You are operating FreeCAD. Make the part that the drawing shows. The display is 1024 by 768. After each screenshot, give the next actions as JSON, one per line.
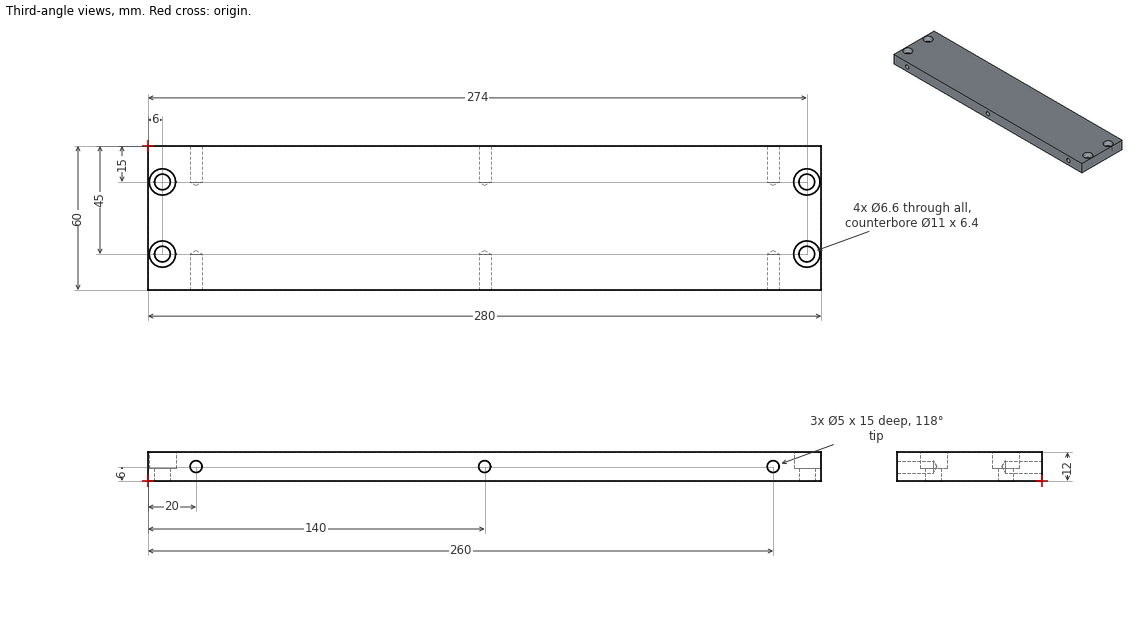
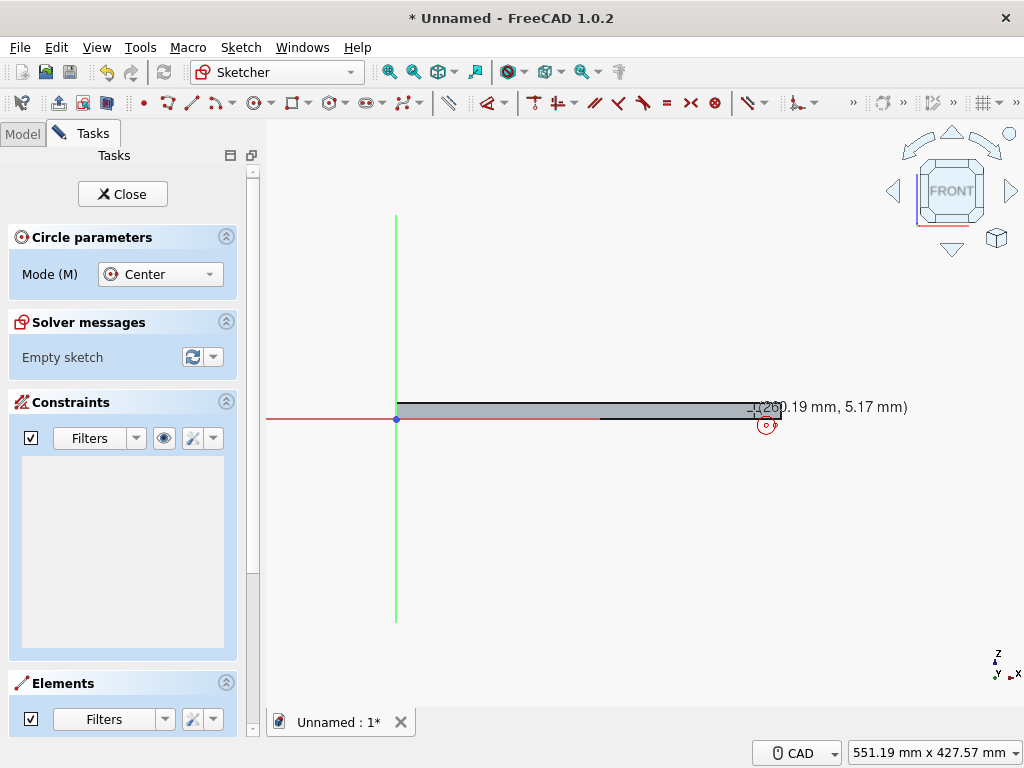
{"action": "scroll", "coordinate": [754, 411], "scroll_direction": "up", "scroll_amount": 4}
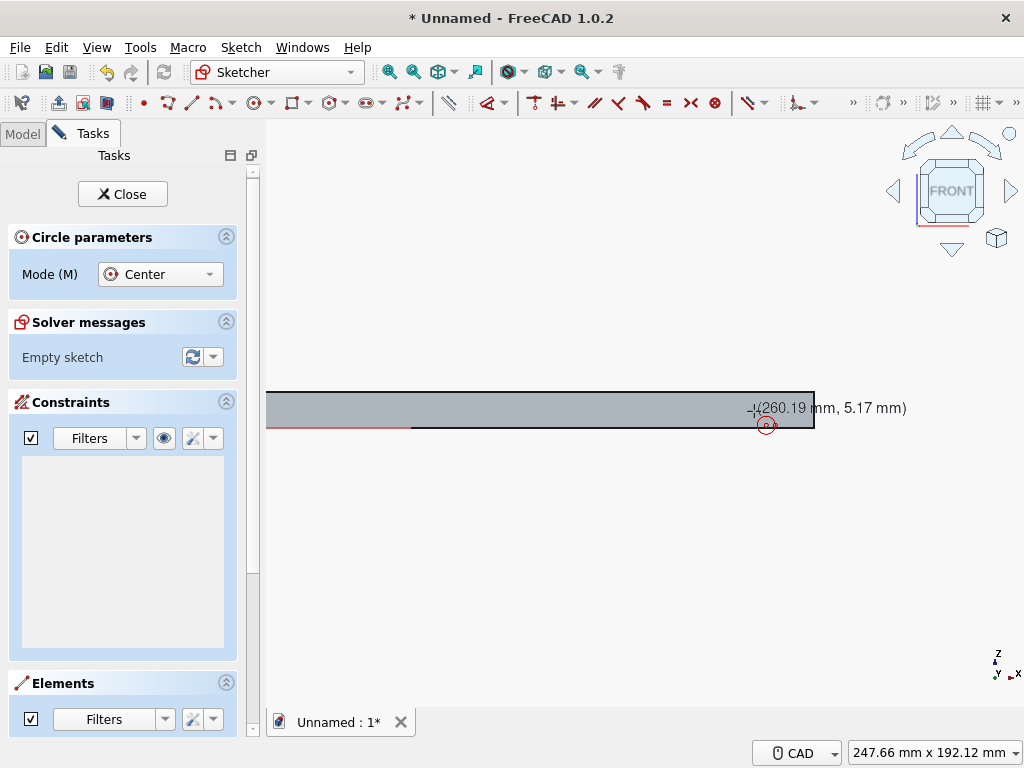
{"action": "left_click", "coordinate": [753, 410]}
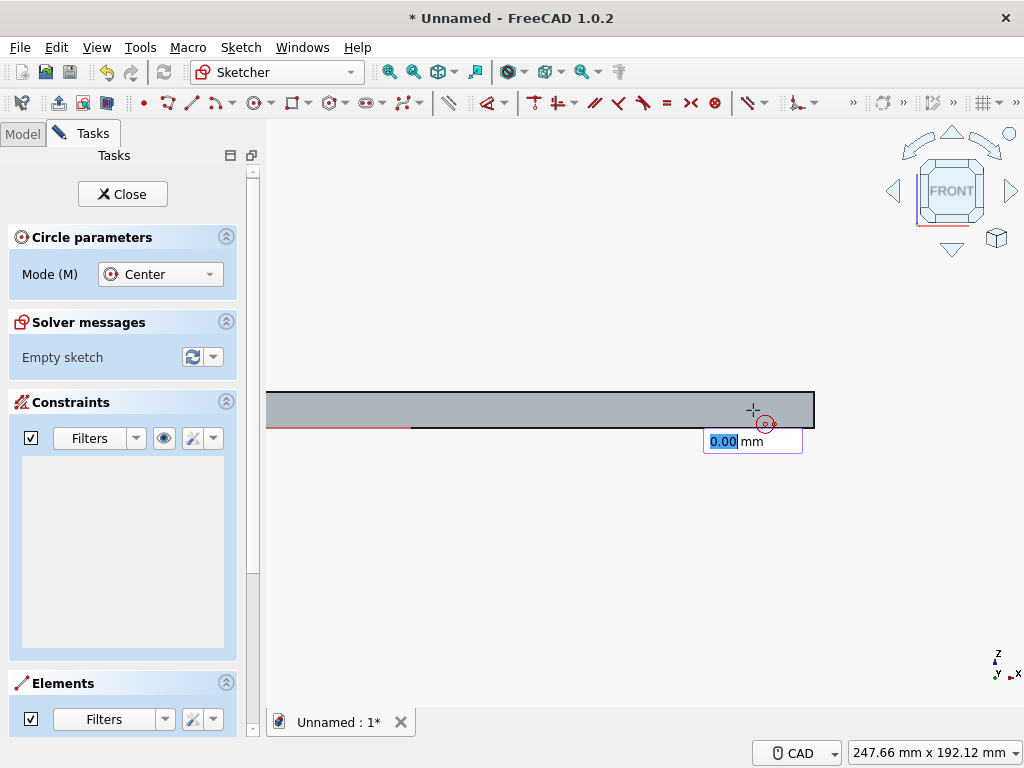
{"action": "scroll", "coordinate": [758, 405], "scroll_direction": "up", "scroll_amount": 4}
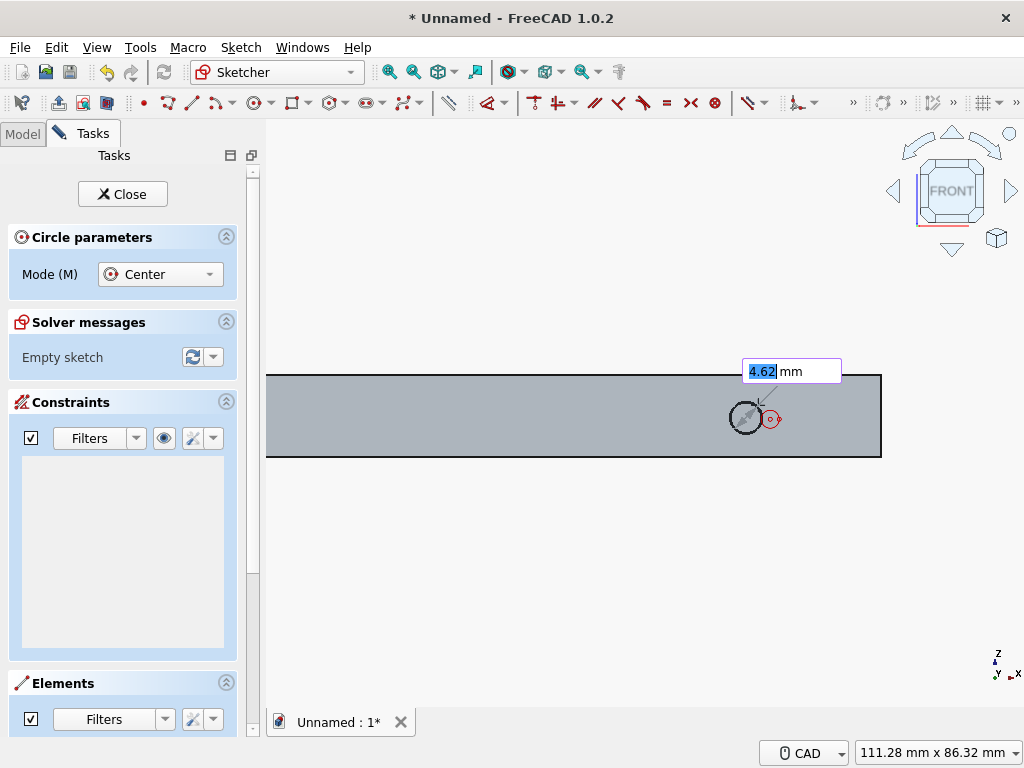
{"action": "left_click", "coordinate": [757, 404]}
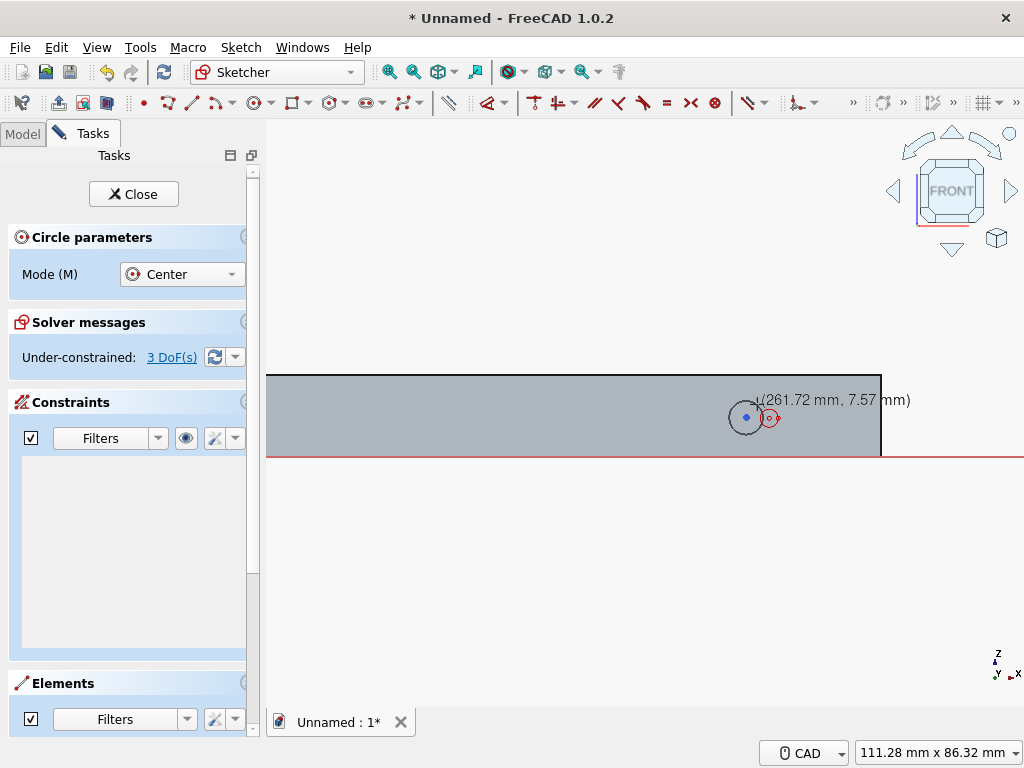
{"action": "scroll", "coordinate": [756, 409], "scroll_direction": "down", "scroll_amount": 8}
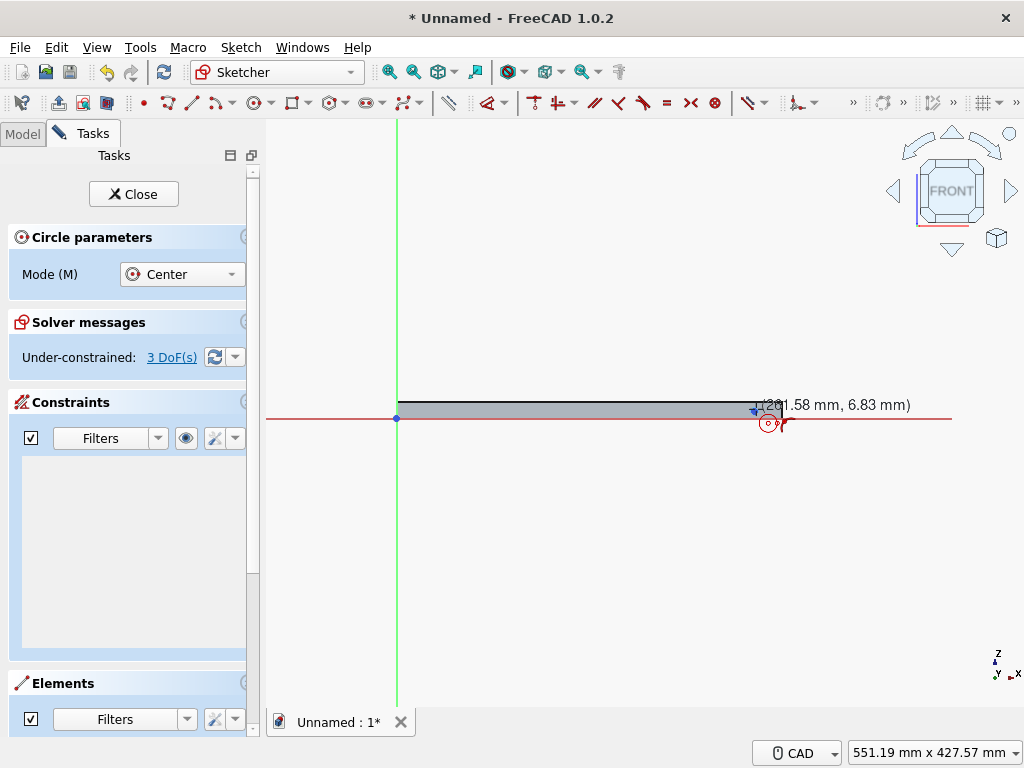
{"action": "scroll", "coordinate": [589, 411], "scroll_direction": "up", "scroll_amount": 10}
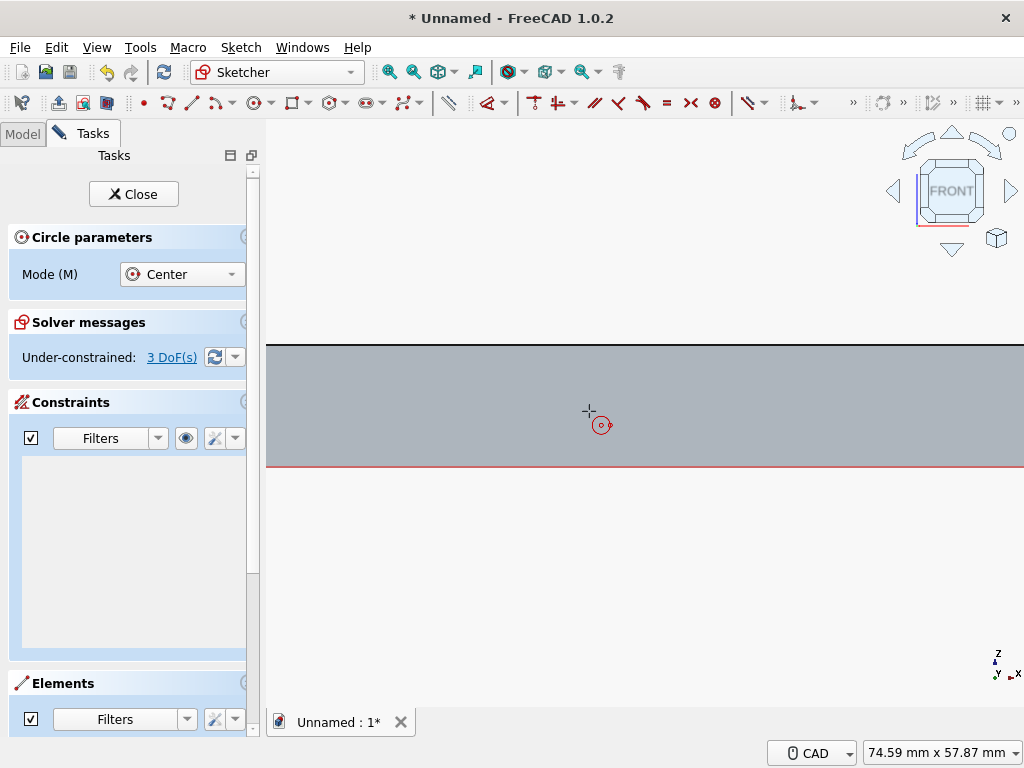
{"action": "scroll", "coordinate": [589, 411], "scroll_direction": "down", "scroll_amount": 10}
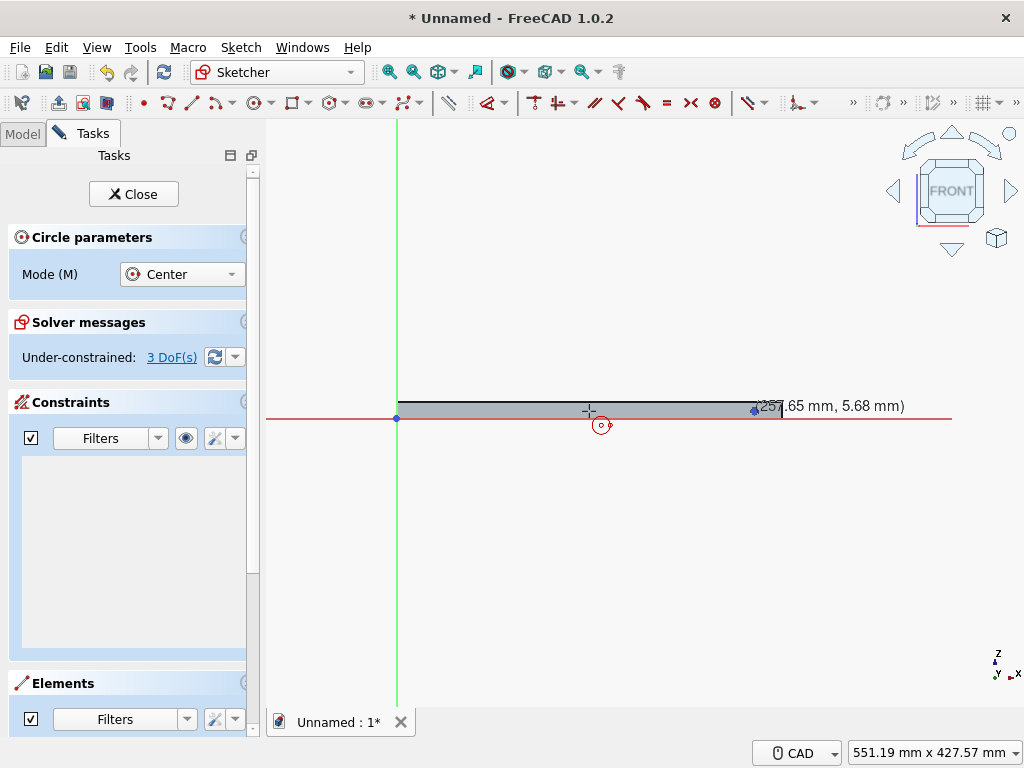
{"action": "scroll", "coordinate": [589, 411], "scroll_direction": "up", "scroll_amount": 4}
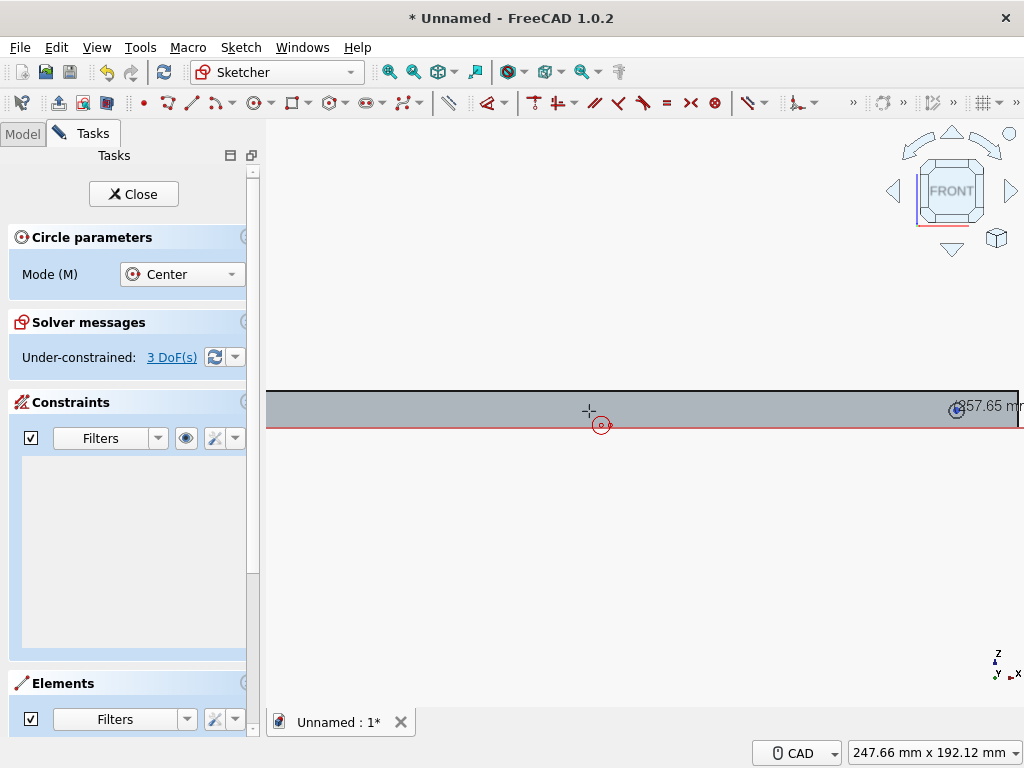
{"action": "left_click", "coordinate": [589, 410]}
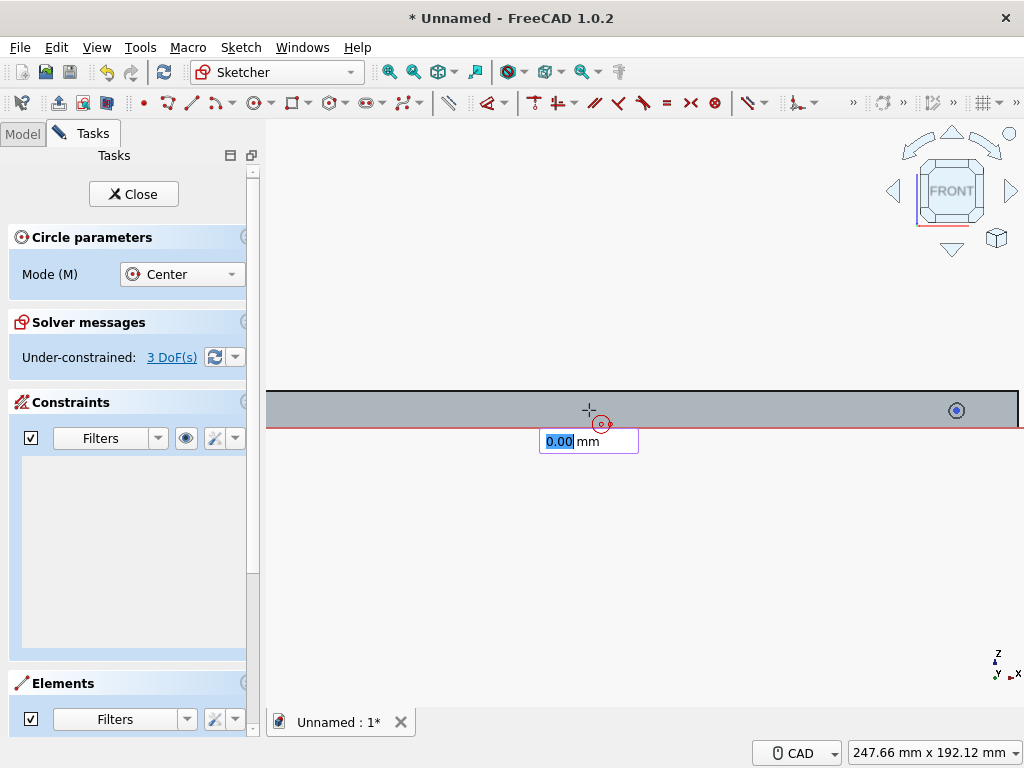
{"action": "scroll", "coordinate": [595, 404], "scroll_direction": "up", "scroll_amount": 4}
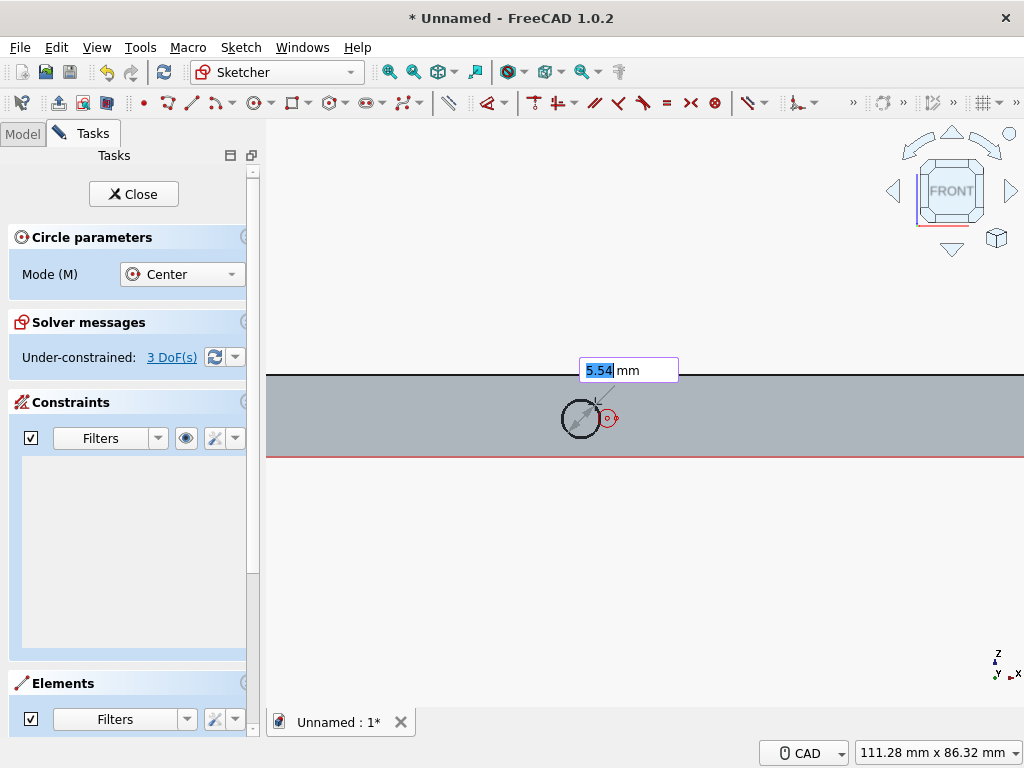
{"action": "left_click", "coordinate": [594, 404]}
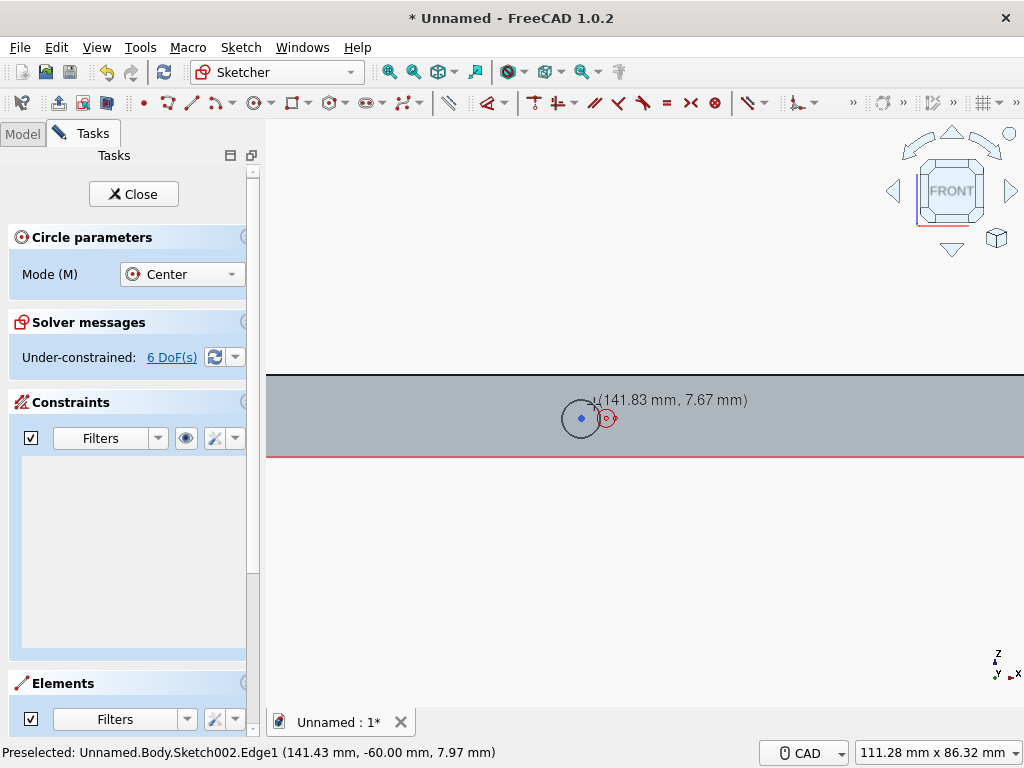
{"action": "scroll", "coordinate": [590, 409], "scroll_direction": "down", "scroll_amount": 8}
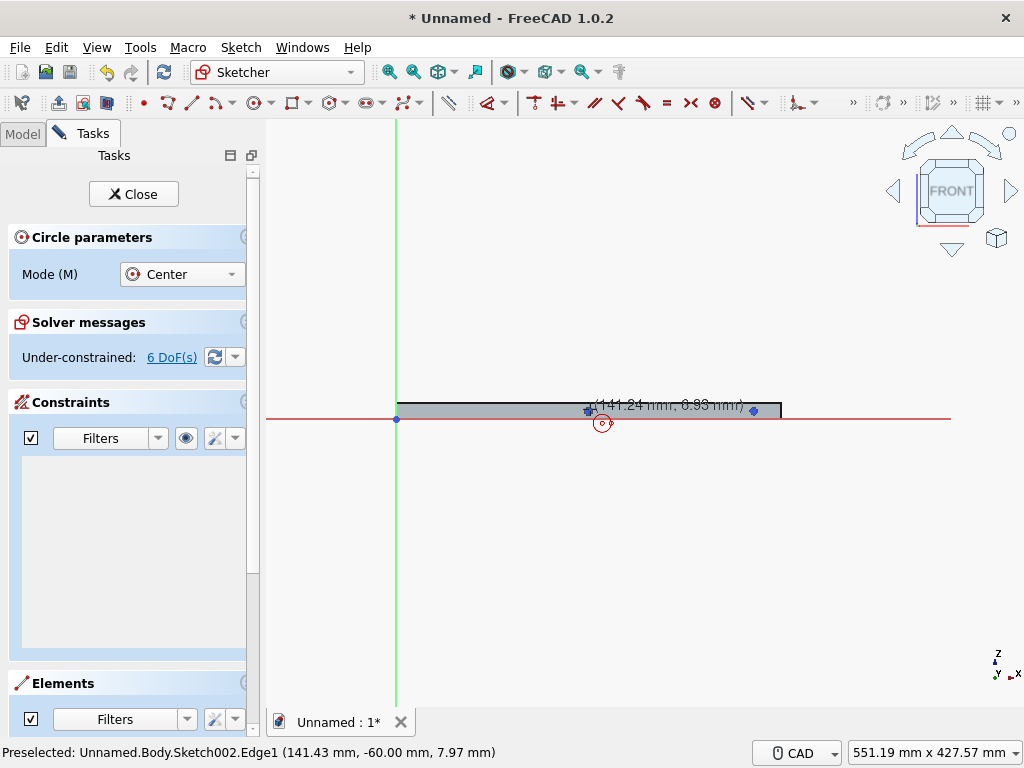
{"action": "scroll", "coordinate": [424, 411], "scroll_direction": "up", "scroll_amount": 10}